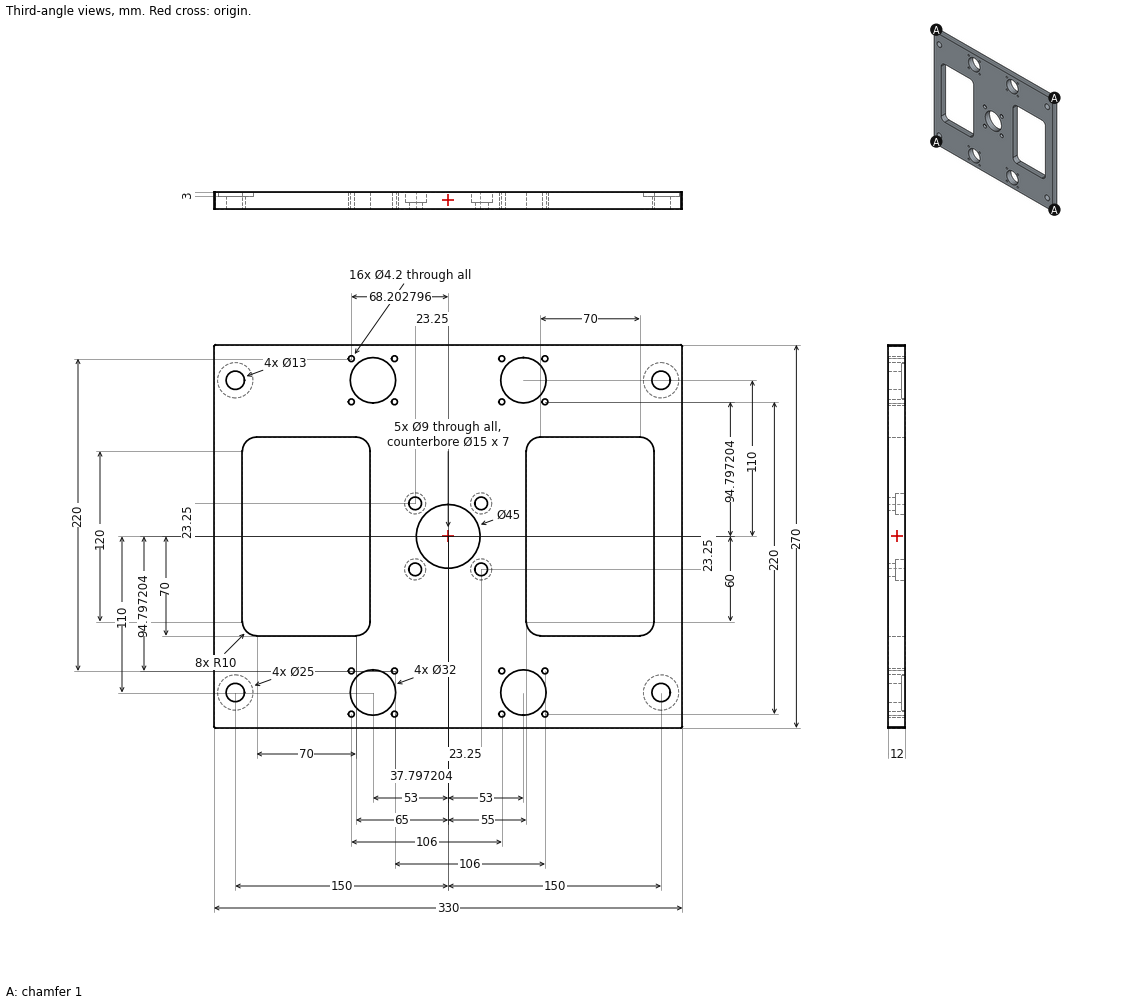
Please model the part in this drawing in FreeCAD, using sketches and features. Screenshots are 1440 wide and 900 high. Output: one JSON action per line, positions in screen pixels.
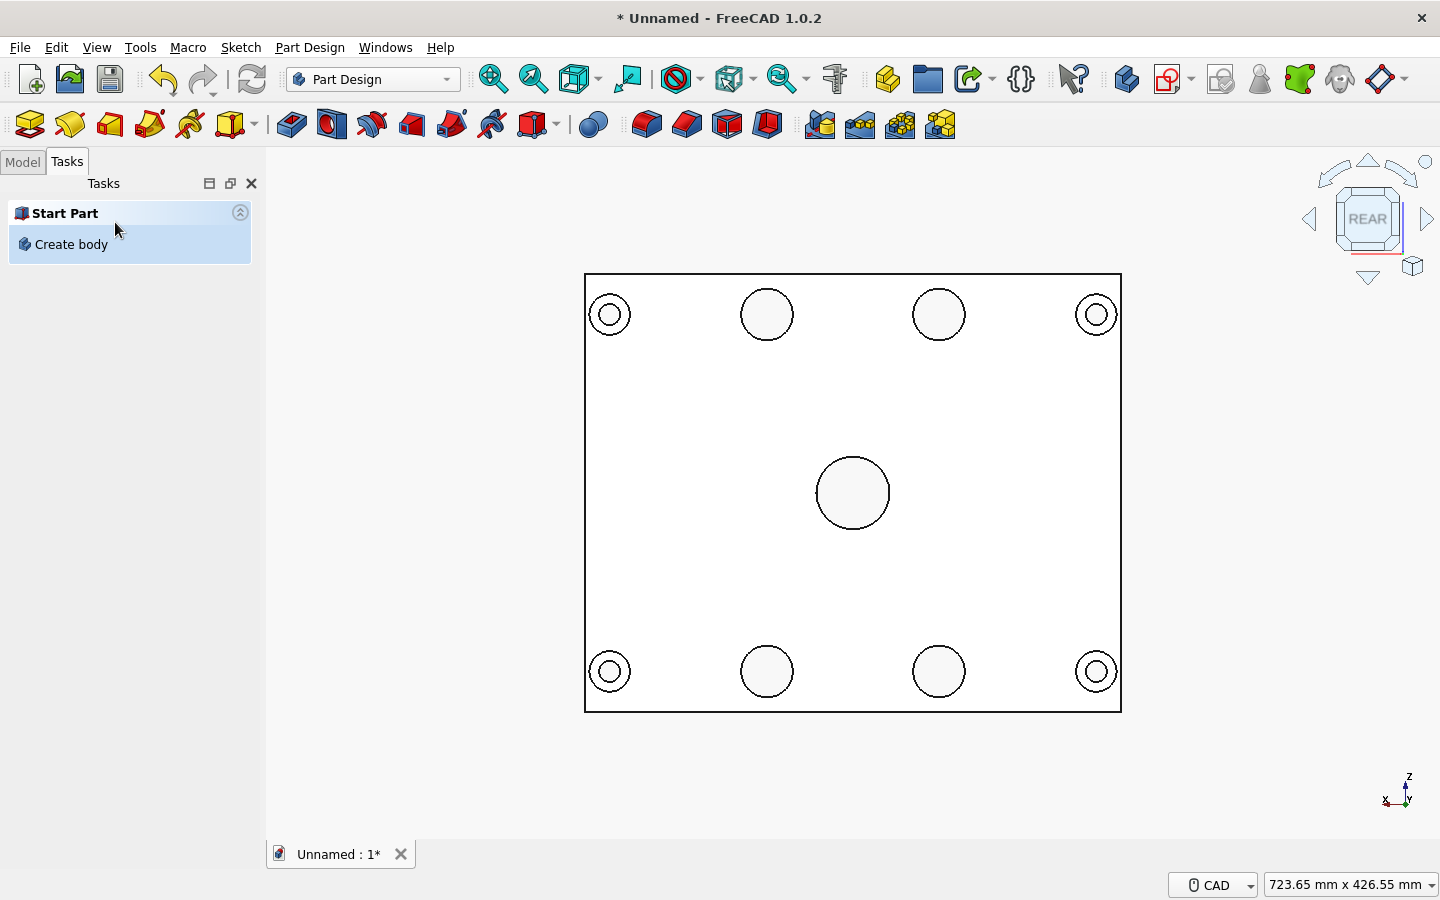
{"action": "left_click", "coordinate": [700, 492]}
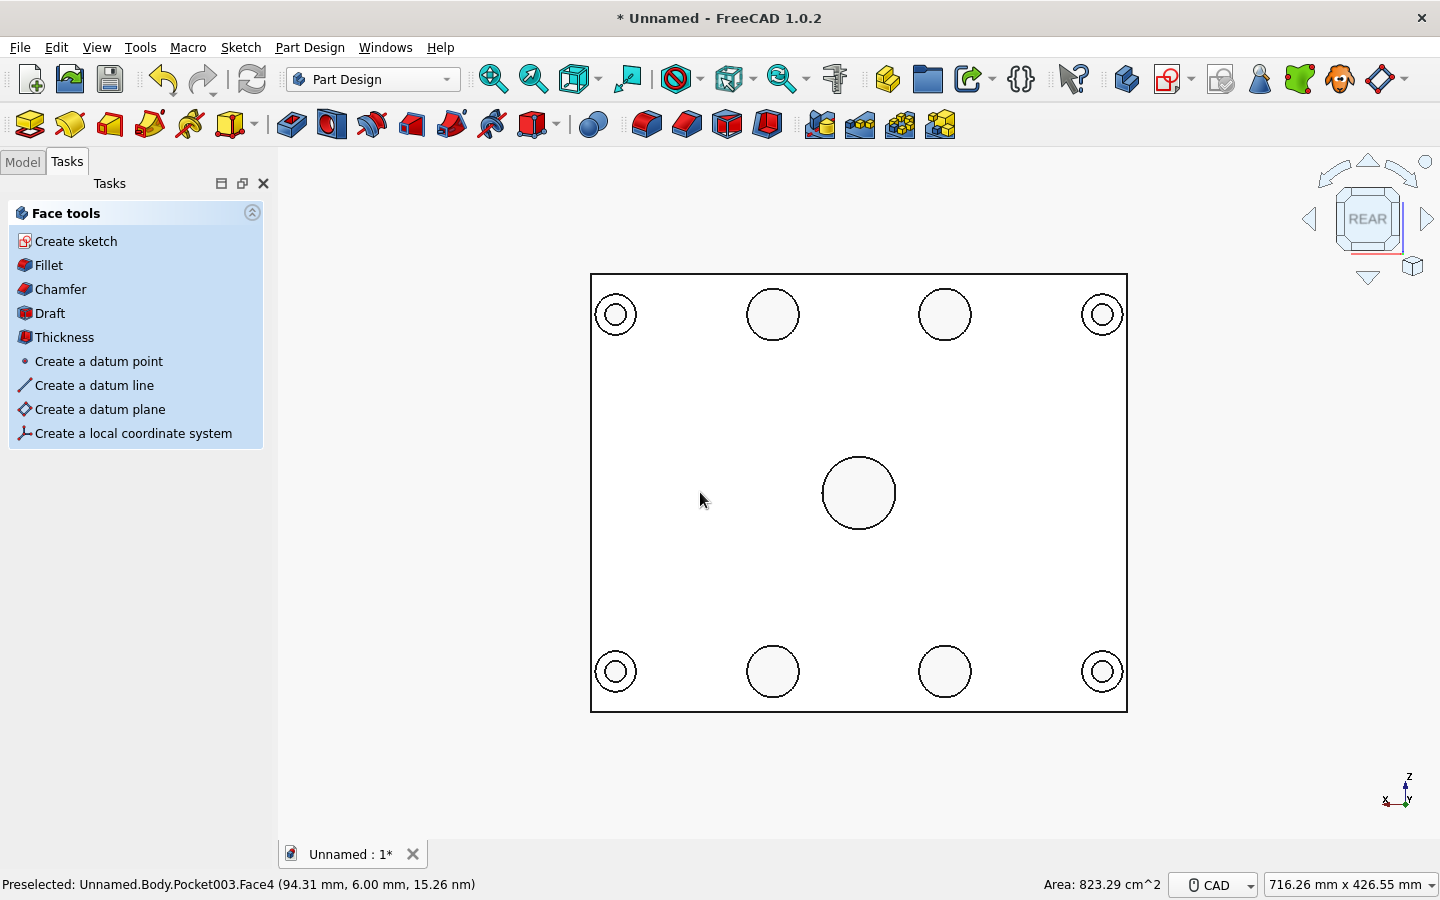
{"action": "left_click", "coordinate": [1168, 80]}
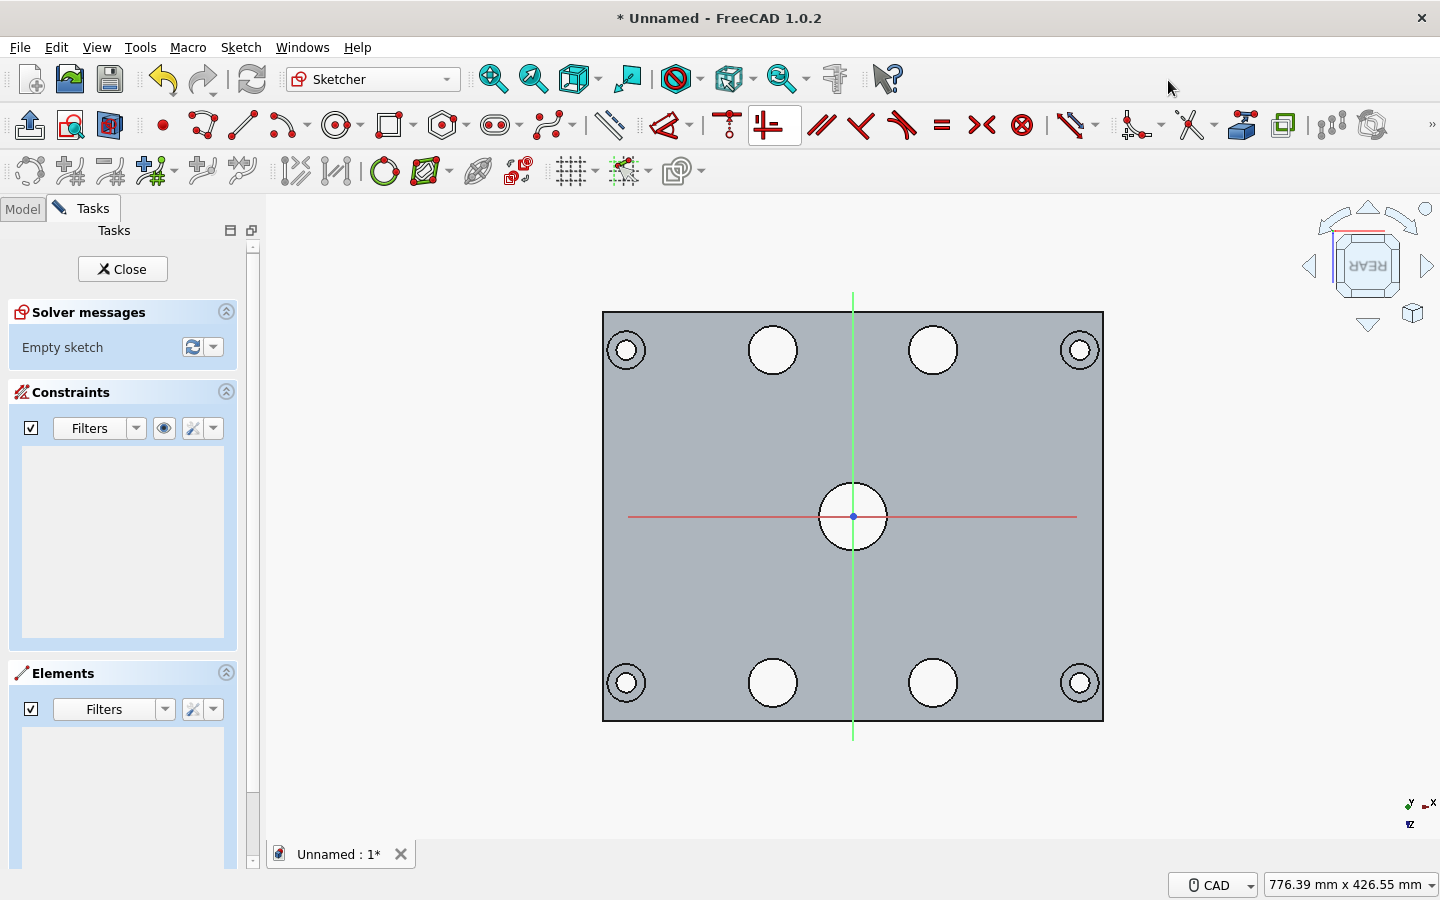
{"action": "key", "text": "g c"}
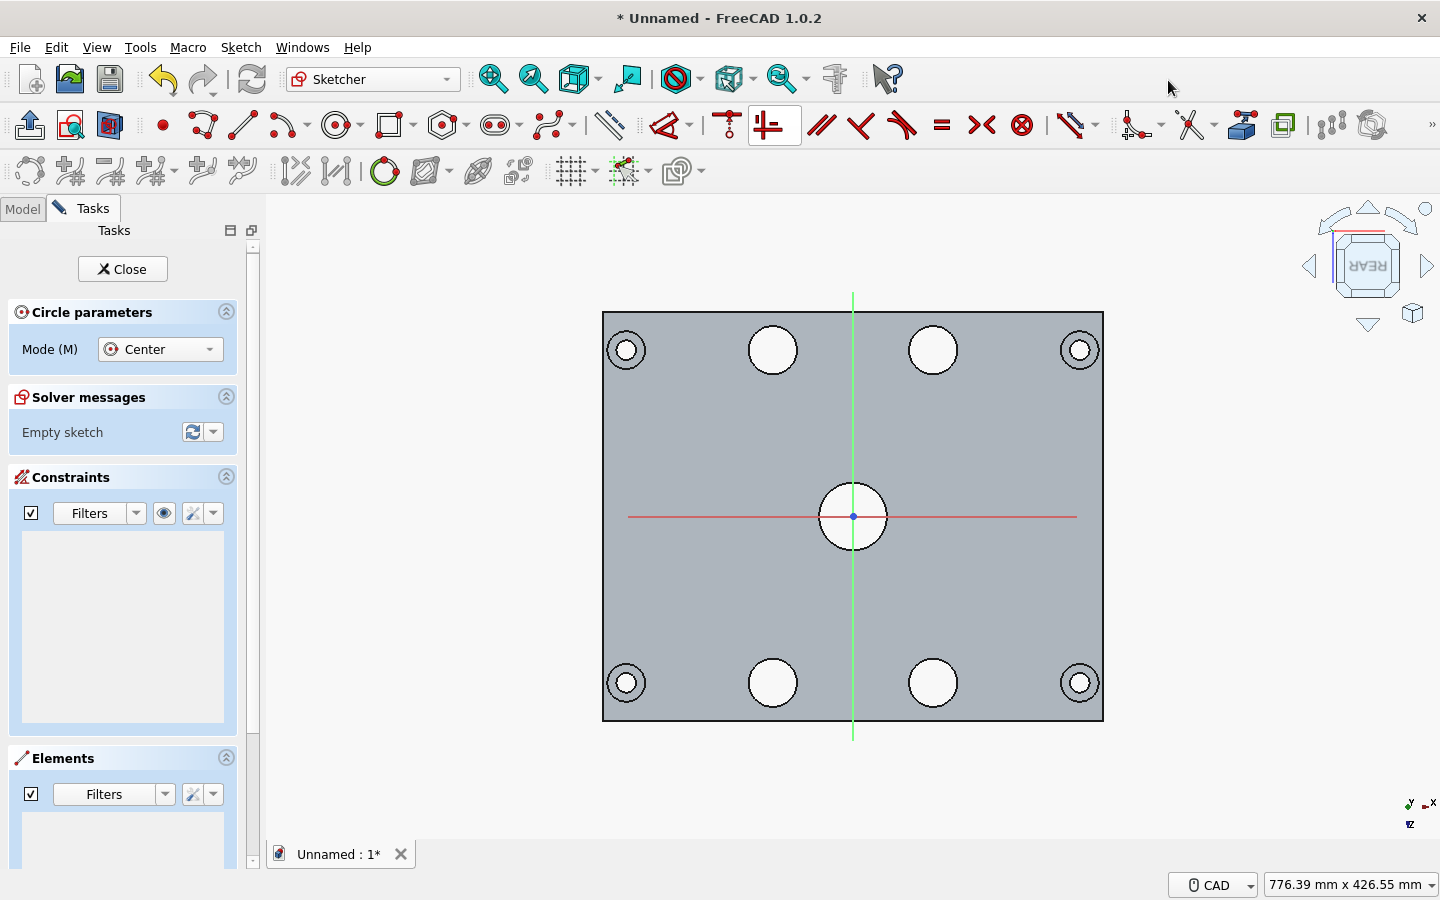
{"action": "scroll", "coordinate": [750, 706], "scroll_direction": "up", "scroll_amount": 10}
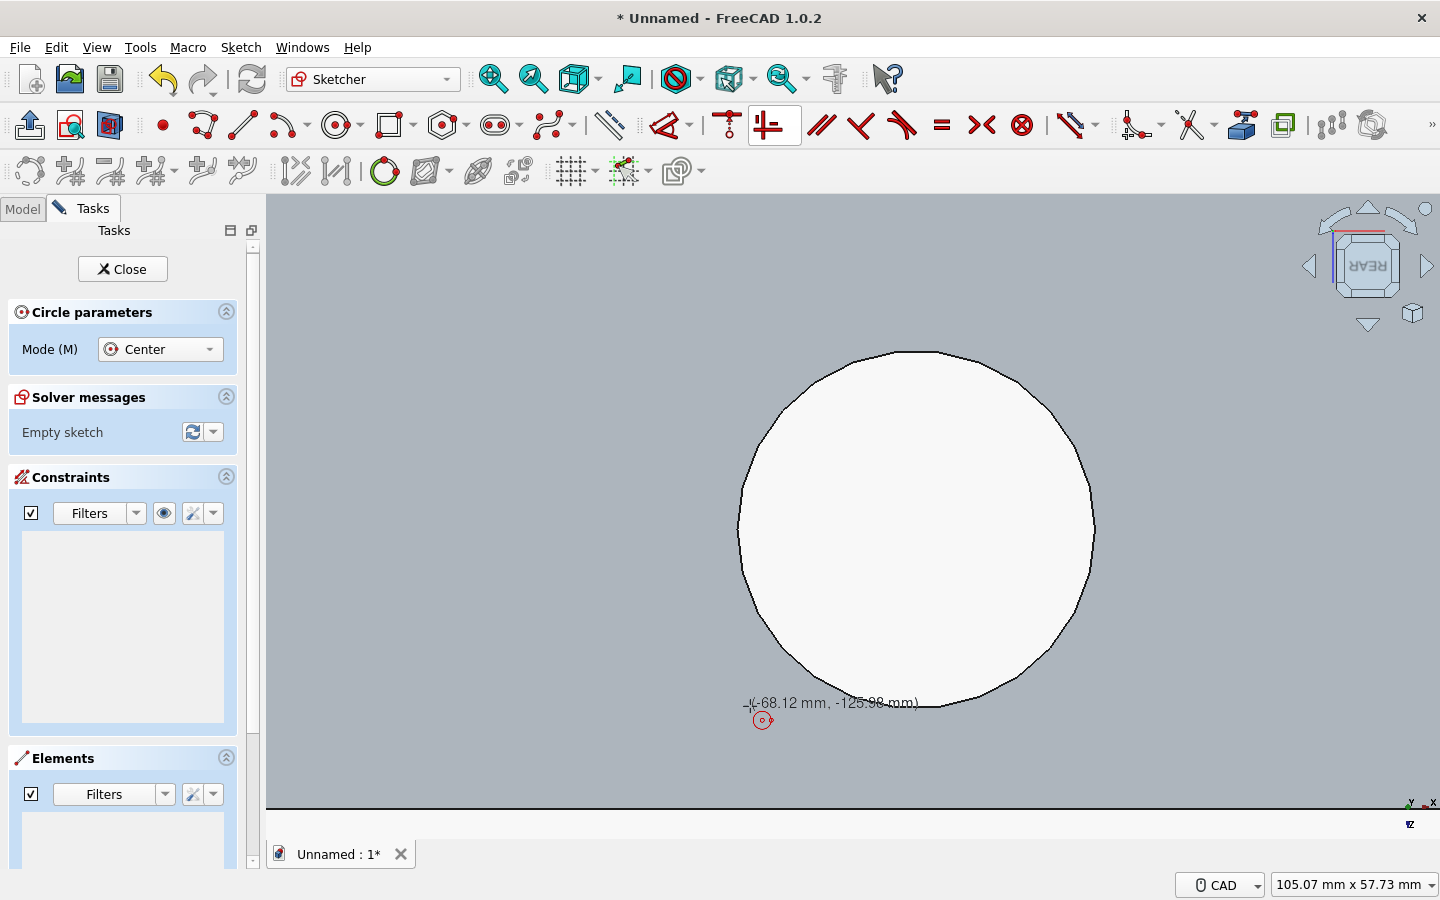
{"action": "scroll", "coordinate": [671, 707], "scroll_direction": "down", "scroll_amount": 10}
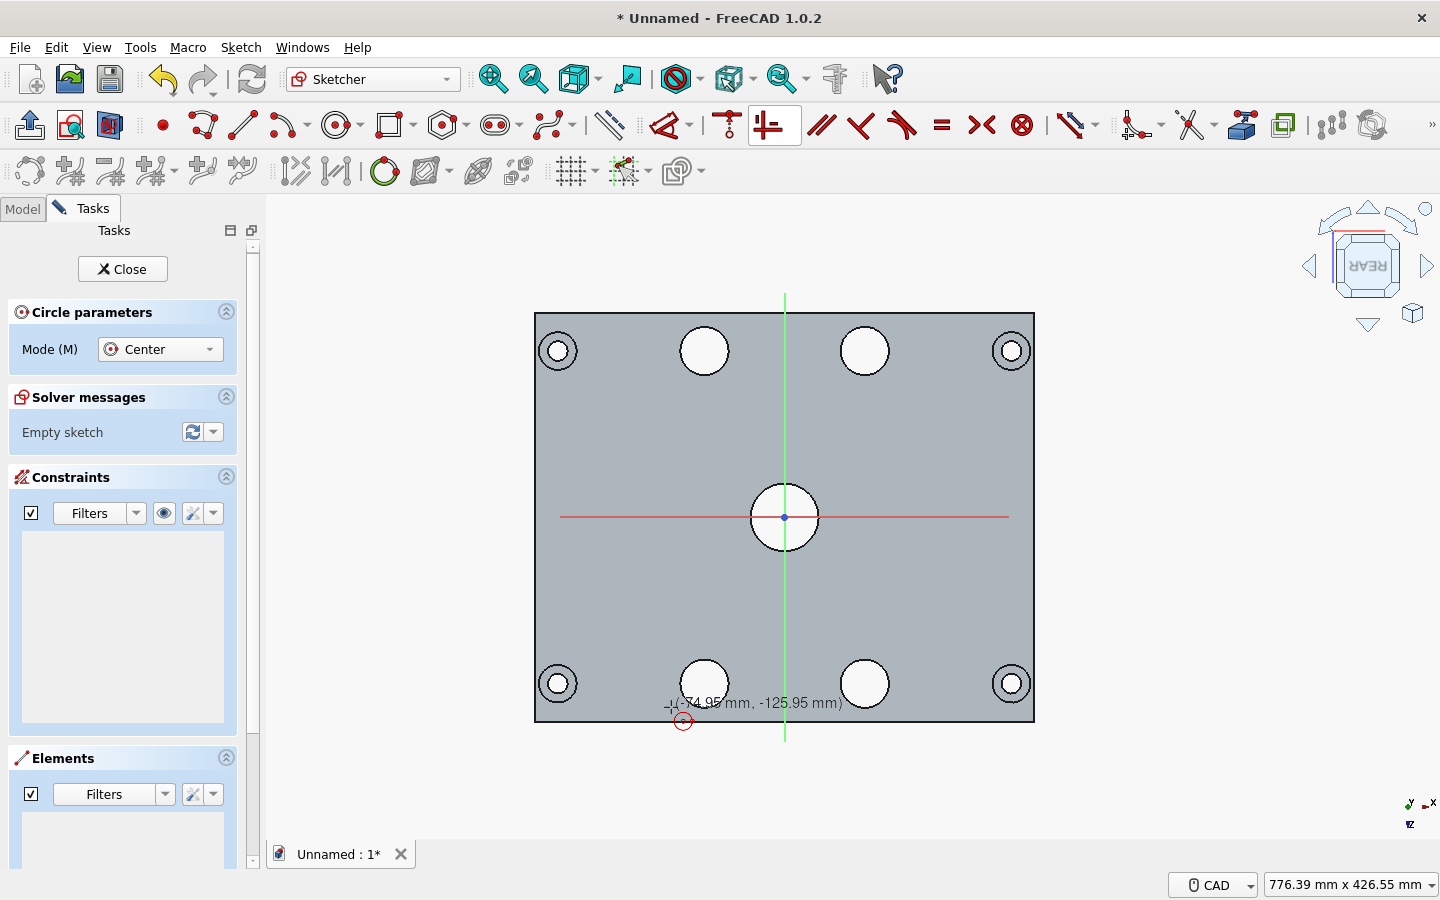
{"action": "left_click", "coordinate": [682, 707]}
{"action": "mouse_move", "coordinate": [684, 704]}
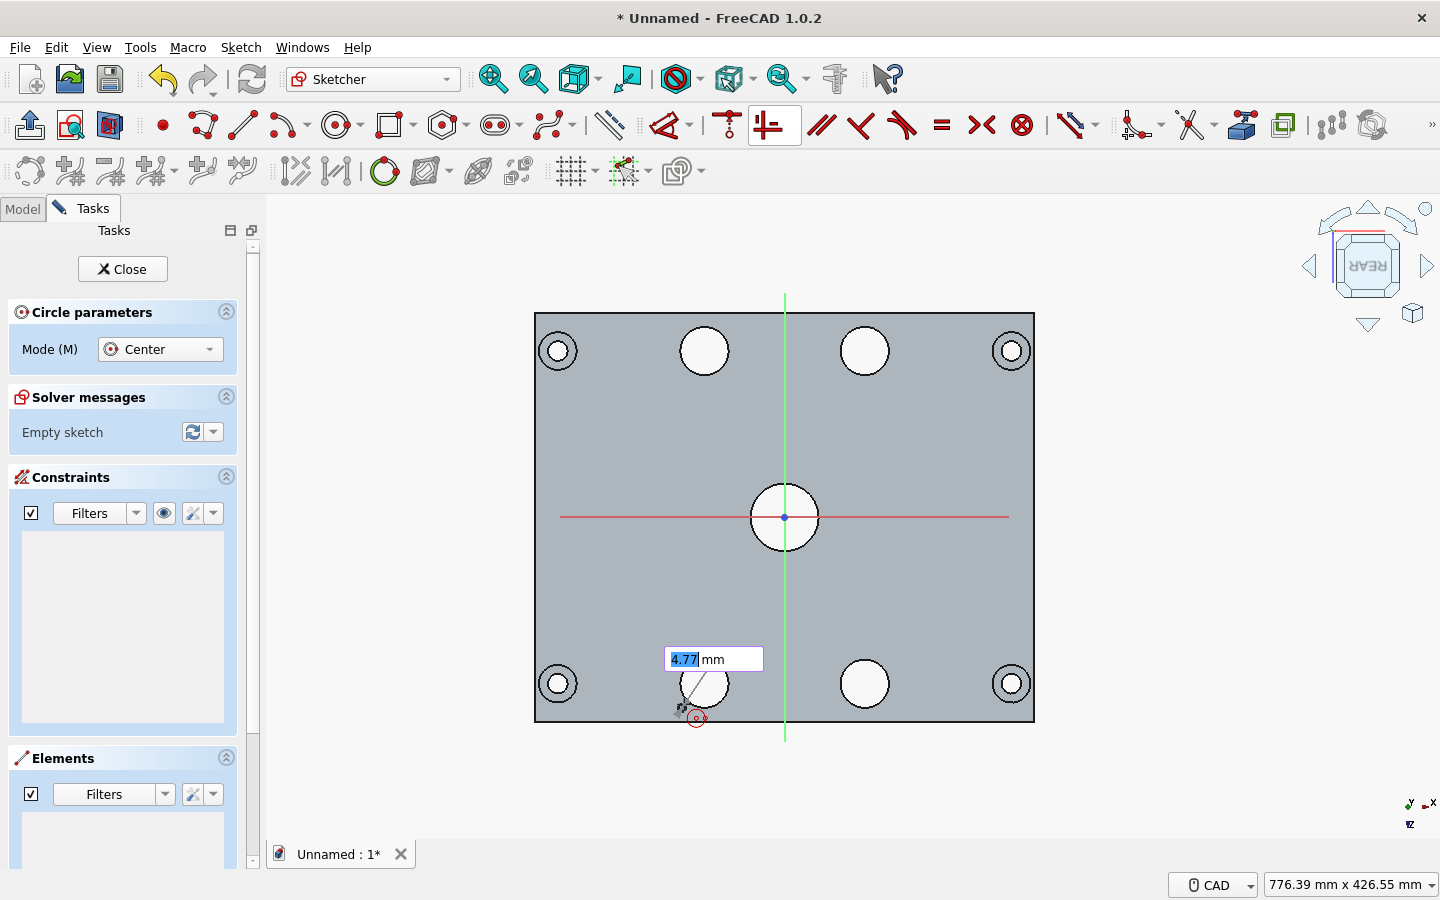
{"action": "type", "text": "4.2"}
{"action": "key", "text": "Return"}